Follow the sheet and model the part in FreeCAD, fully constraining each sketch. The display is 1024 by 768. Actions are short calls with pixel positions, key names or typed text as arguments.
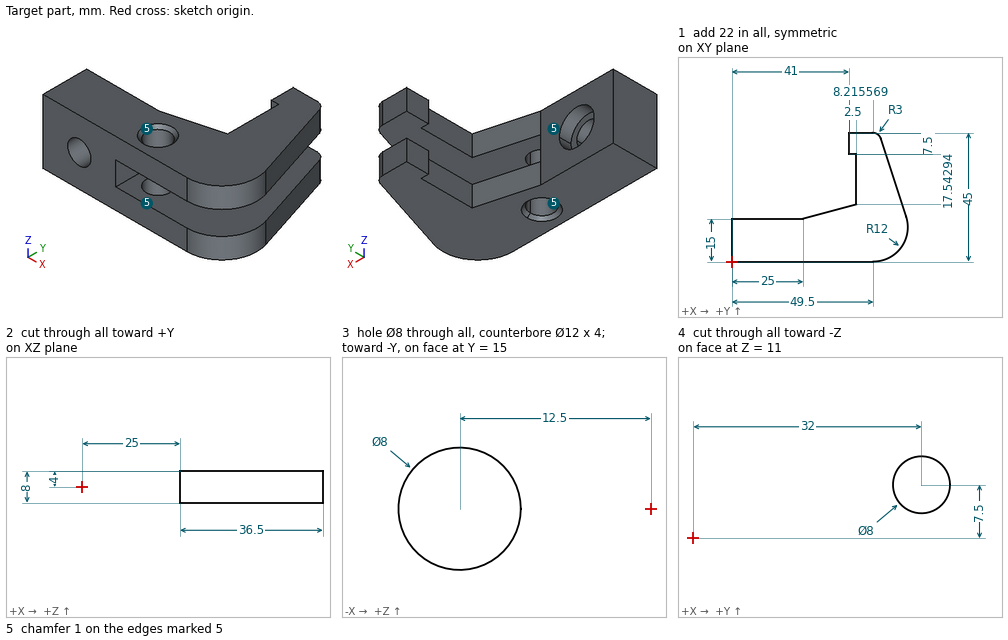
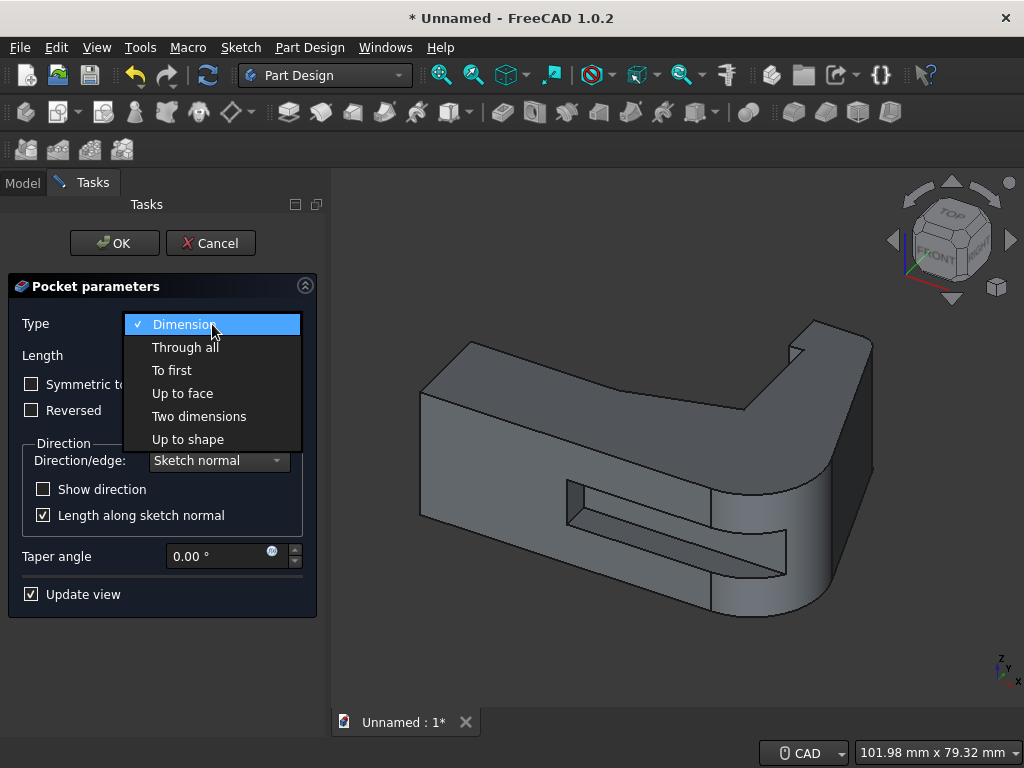
click(212, 348)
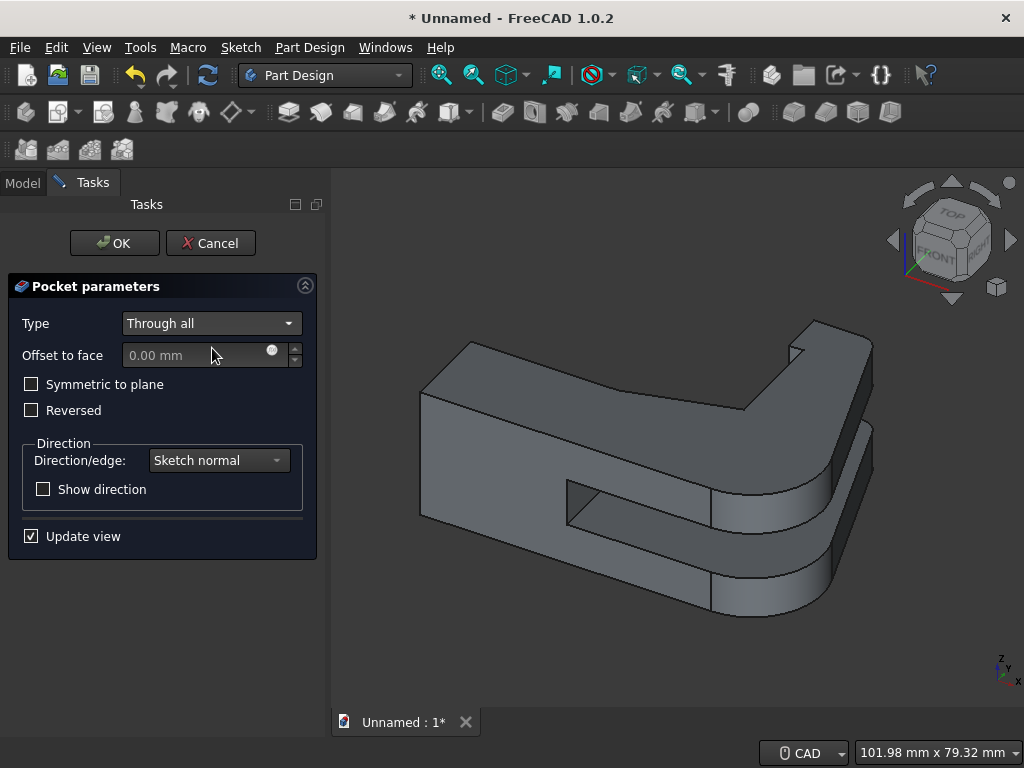
click(115, 243)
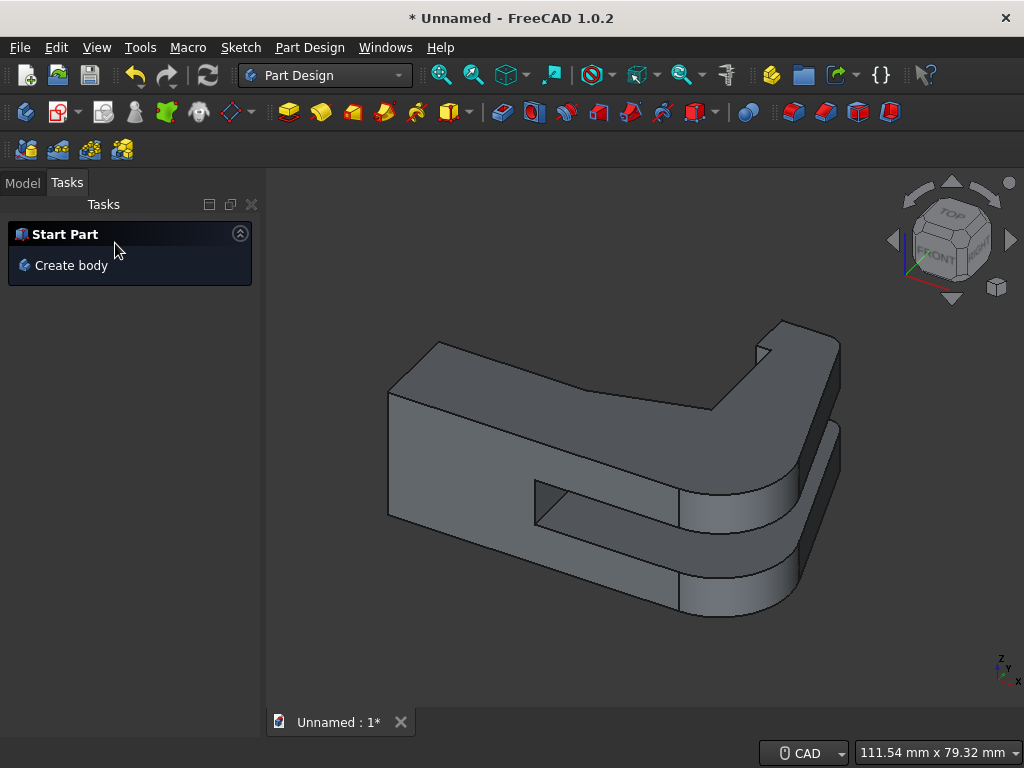
key(4)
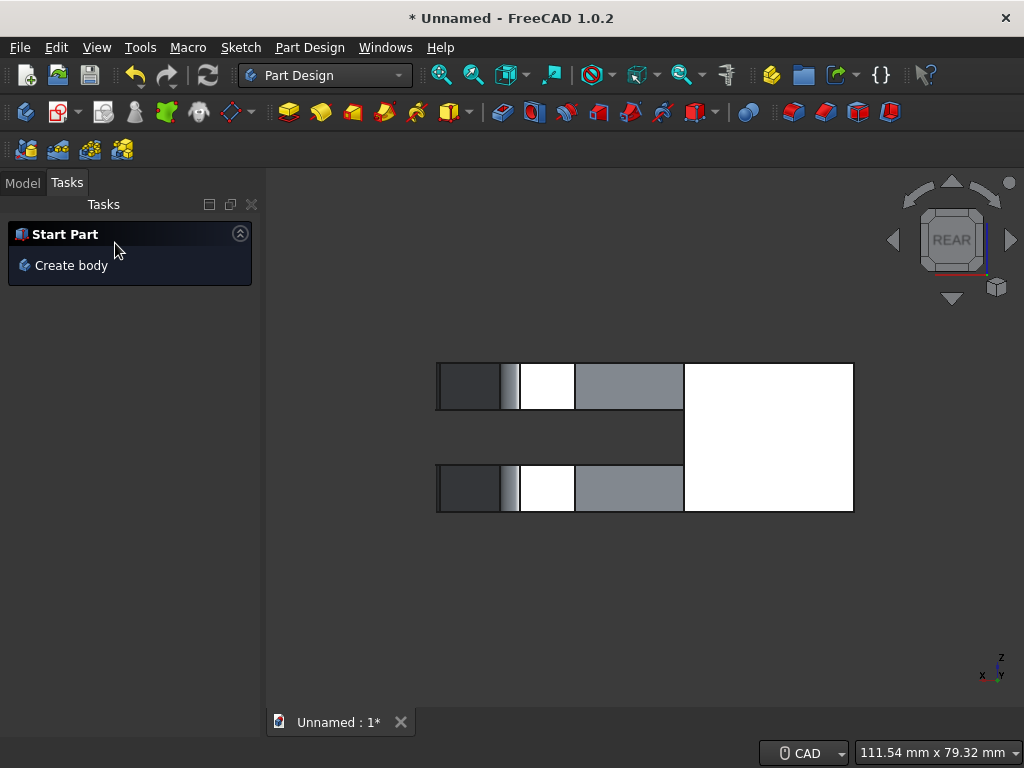
click(769, 436)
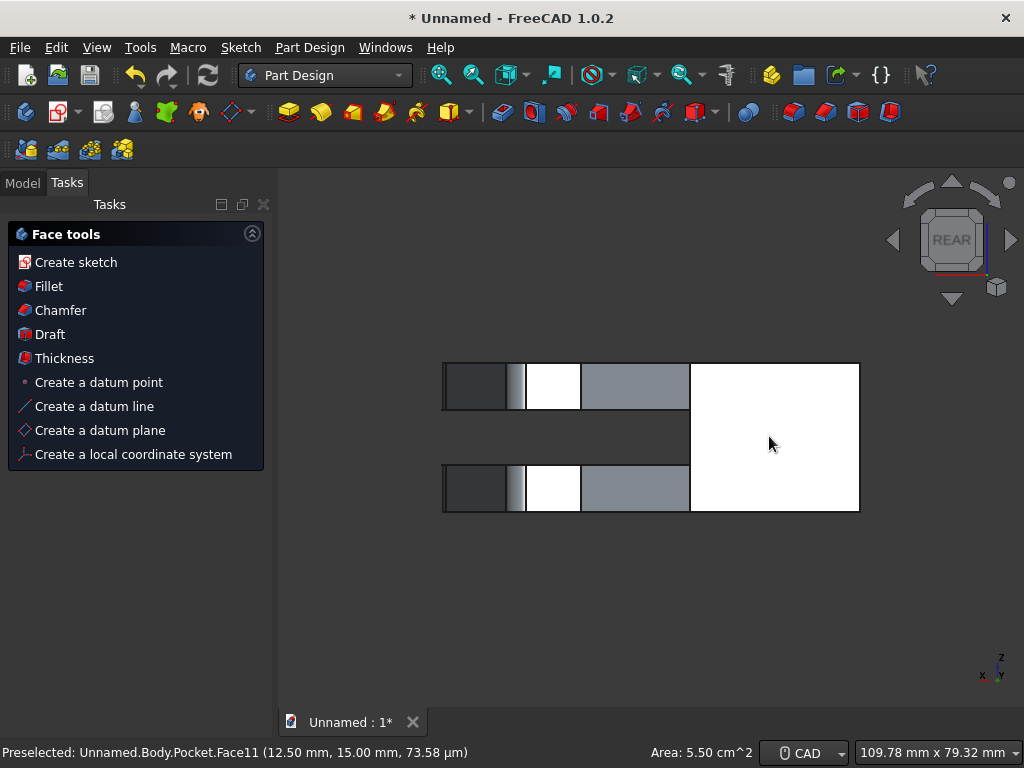
click(58, 112)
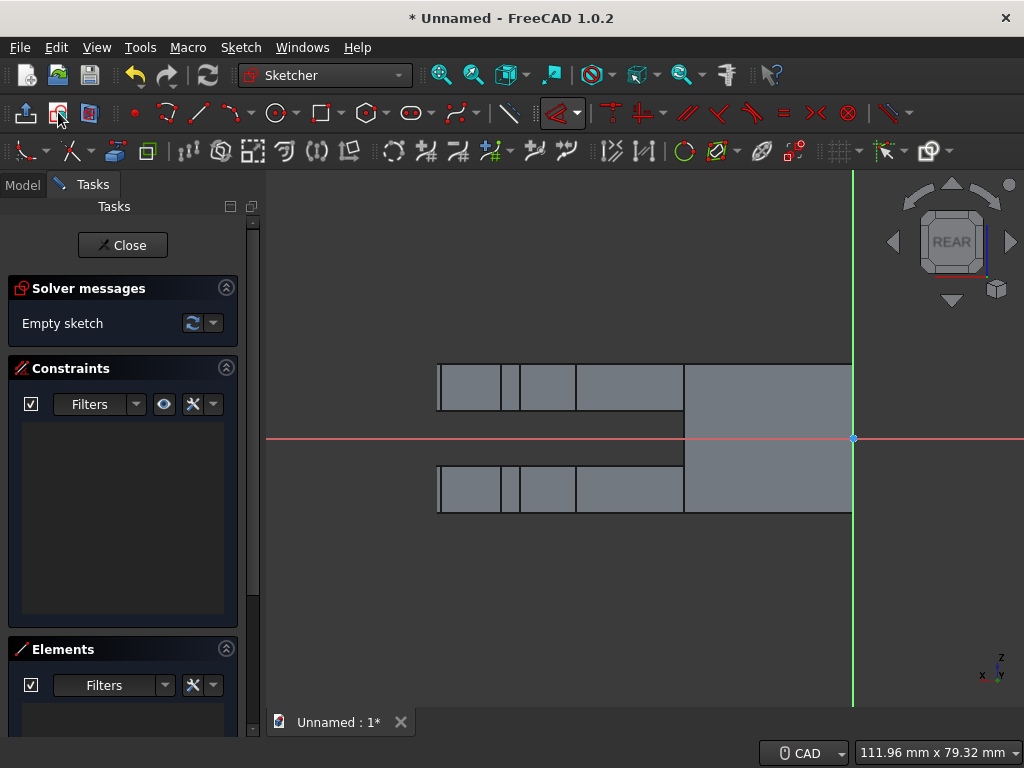
scroll(576, 438, down, 5)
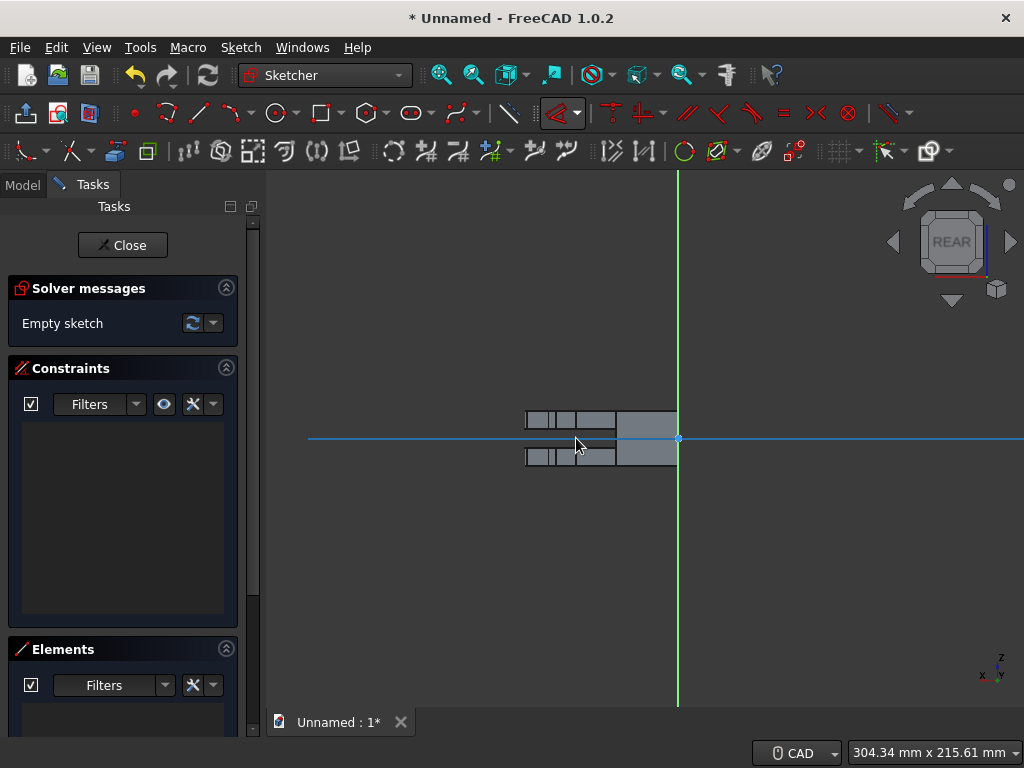
scroll(668, 438, up, 11)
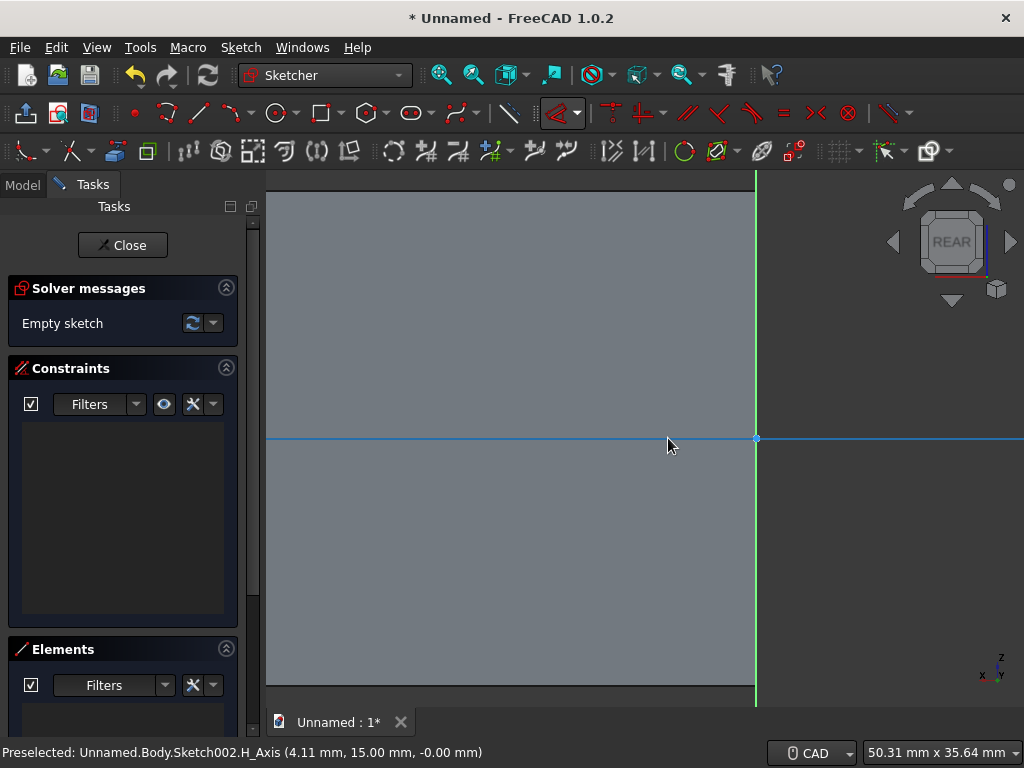
key(g)
key(c)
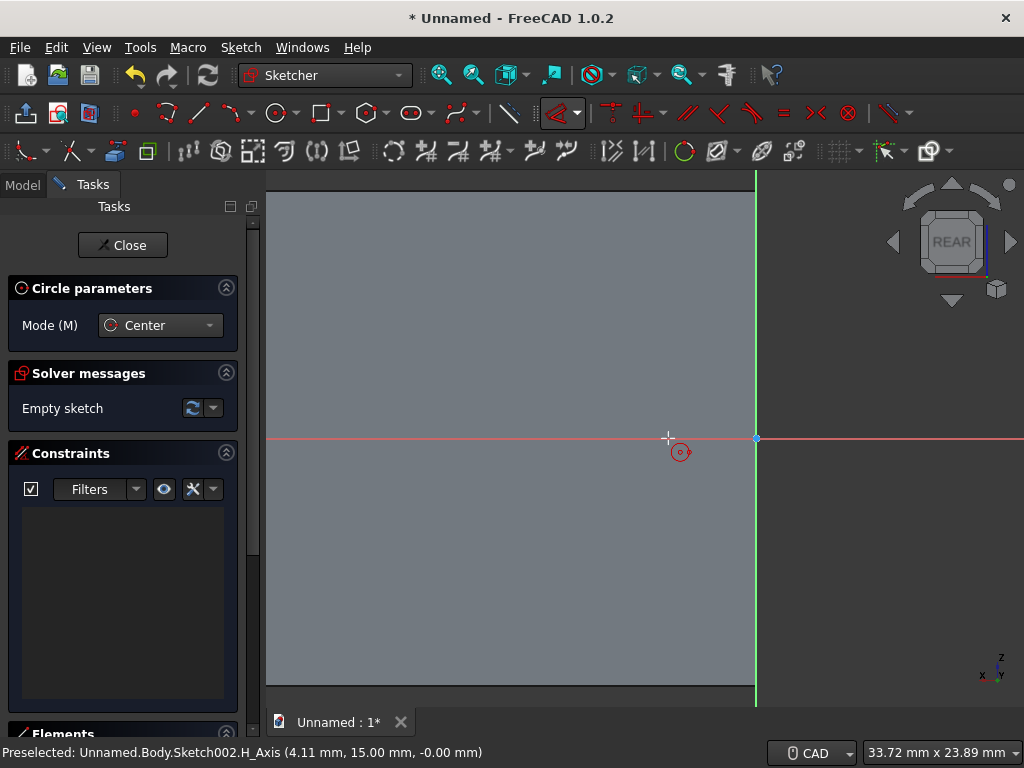
click(475, 438)
click(539, 375)
key(Escape)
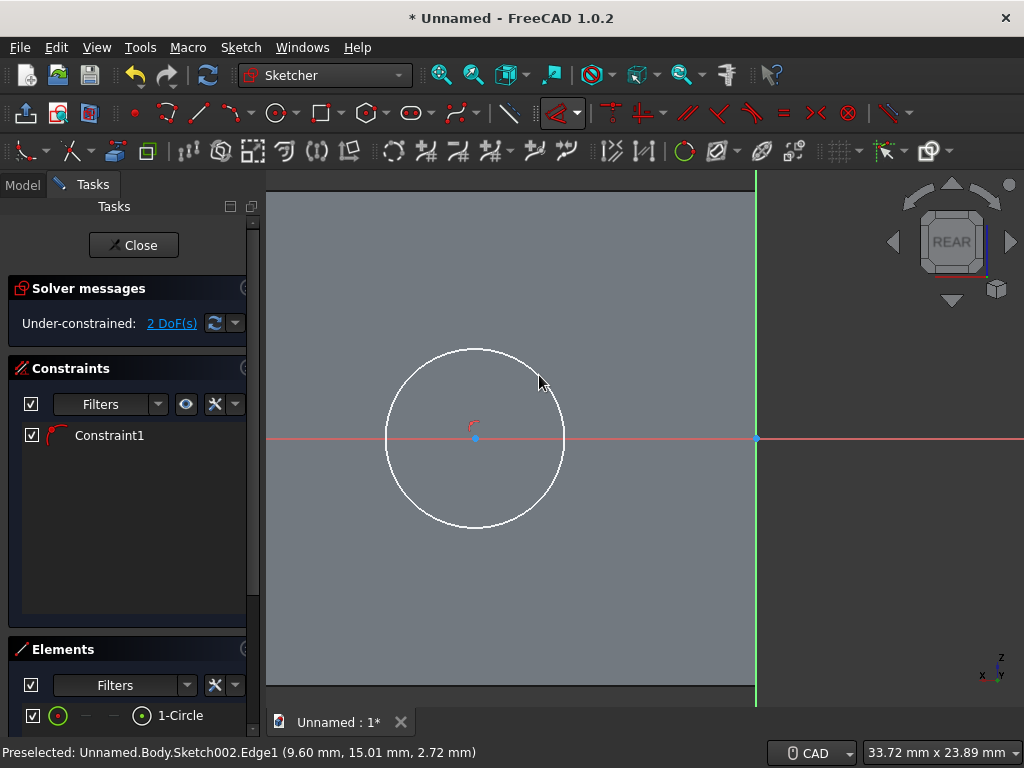
click(538, 375)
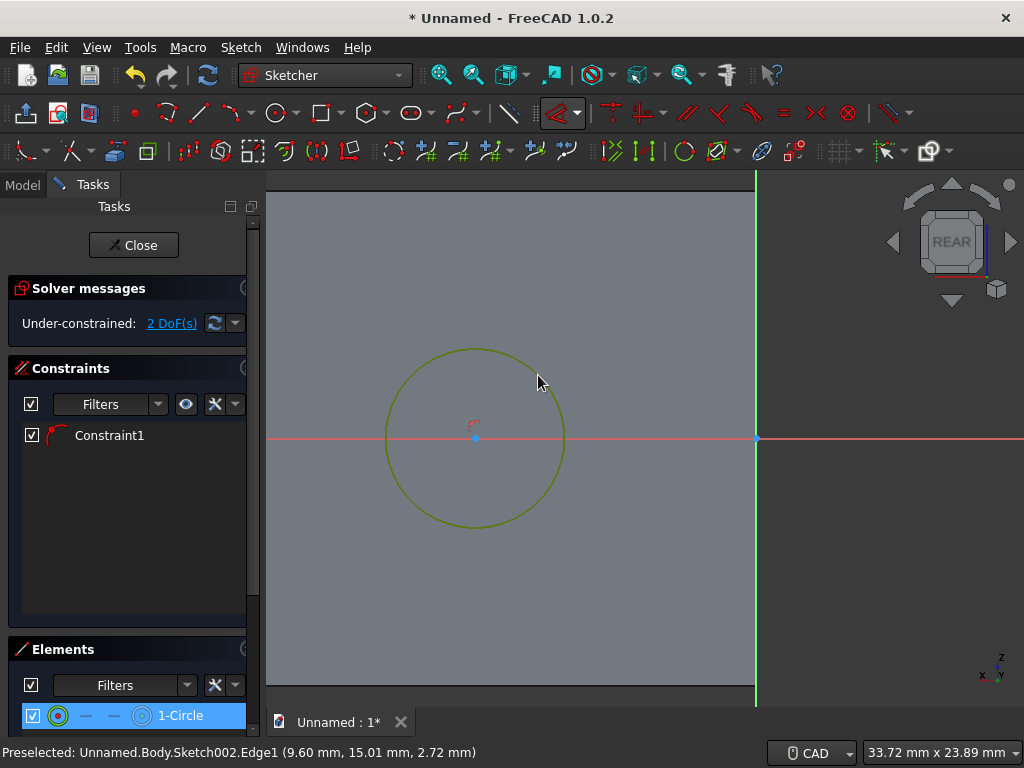
key(k)
key(o)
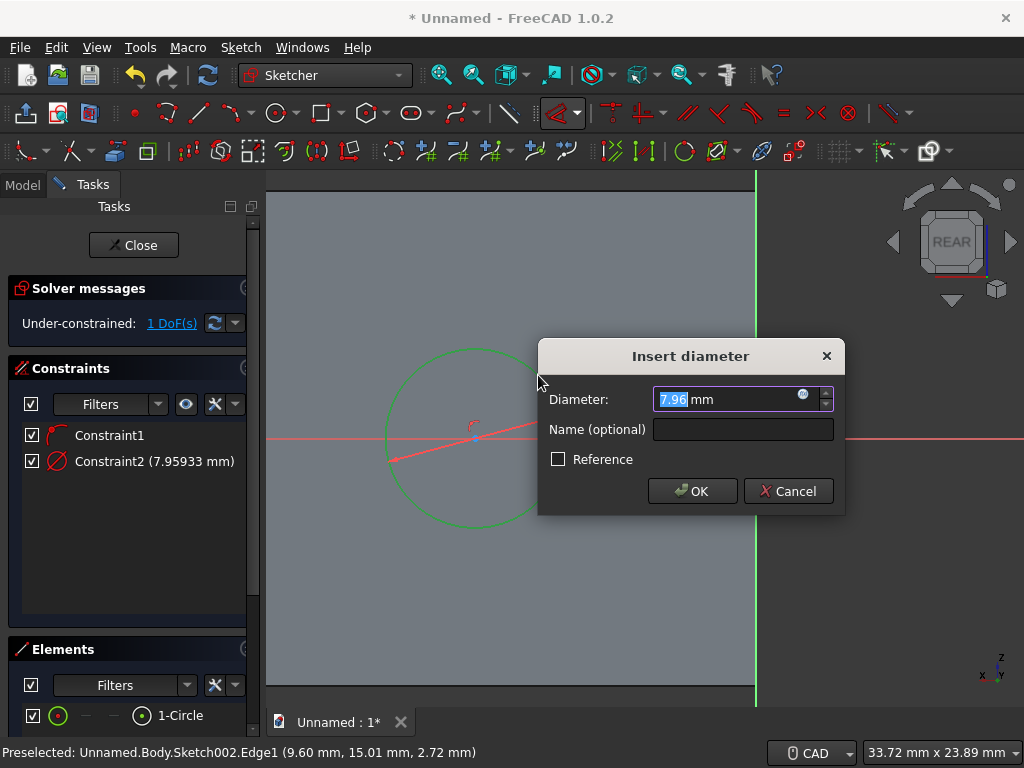
text(8)
key(Return)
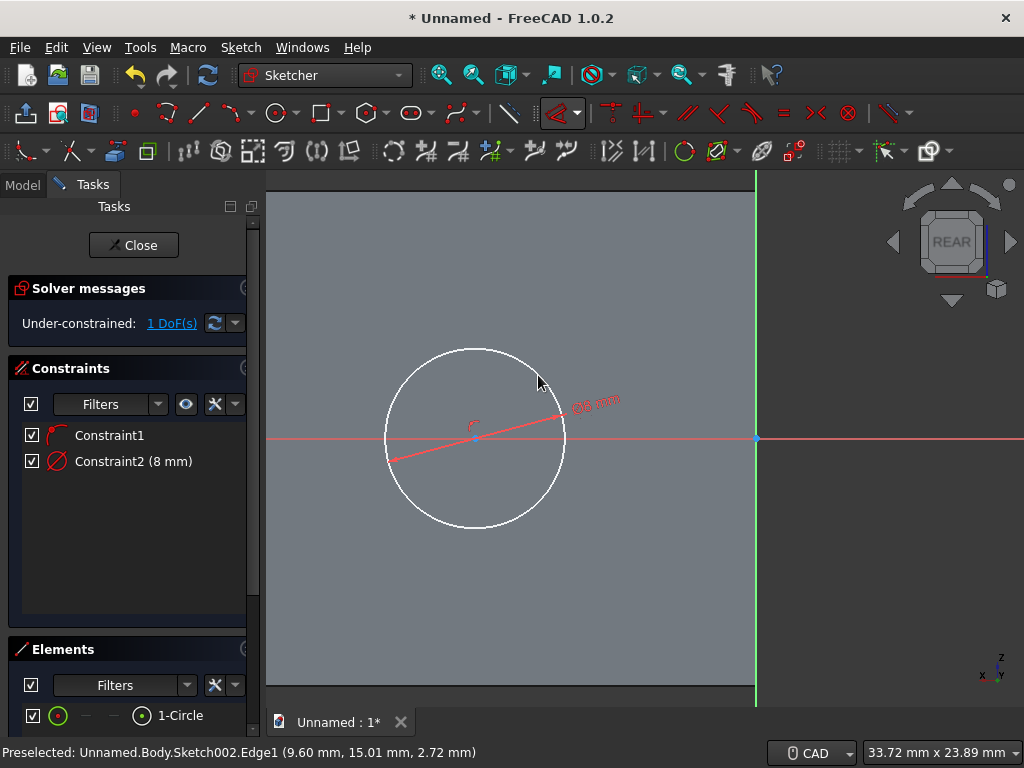
click(475, 438)